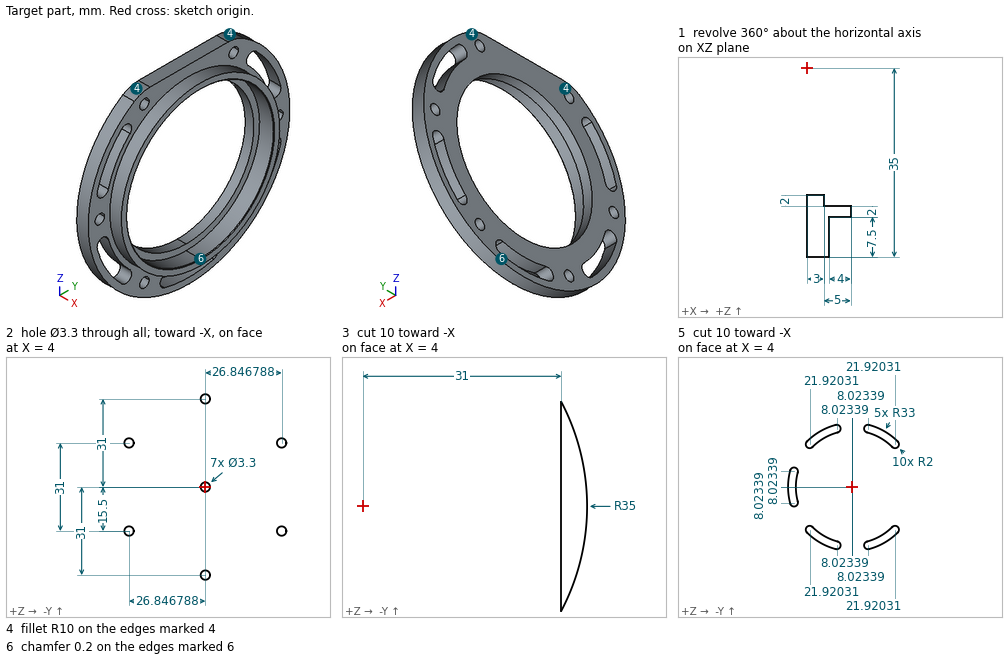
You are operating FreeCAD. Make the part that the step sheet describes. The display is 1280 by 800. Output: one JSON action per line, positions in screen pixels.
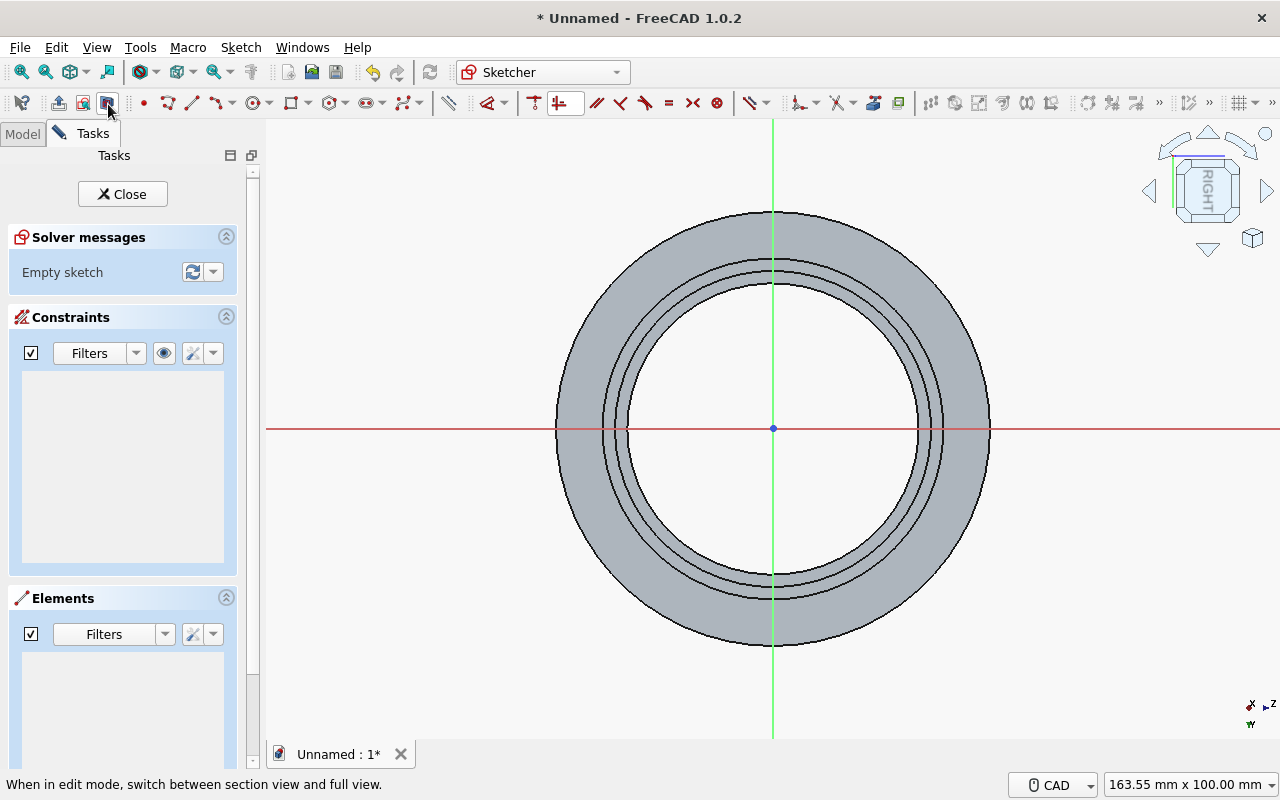
{"action": "left_click", "coordinate": [254, 104]}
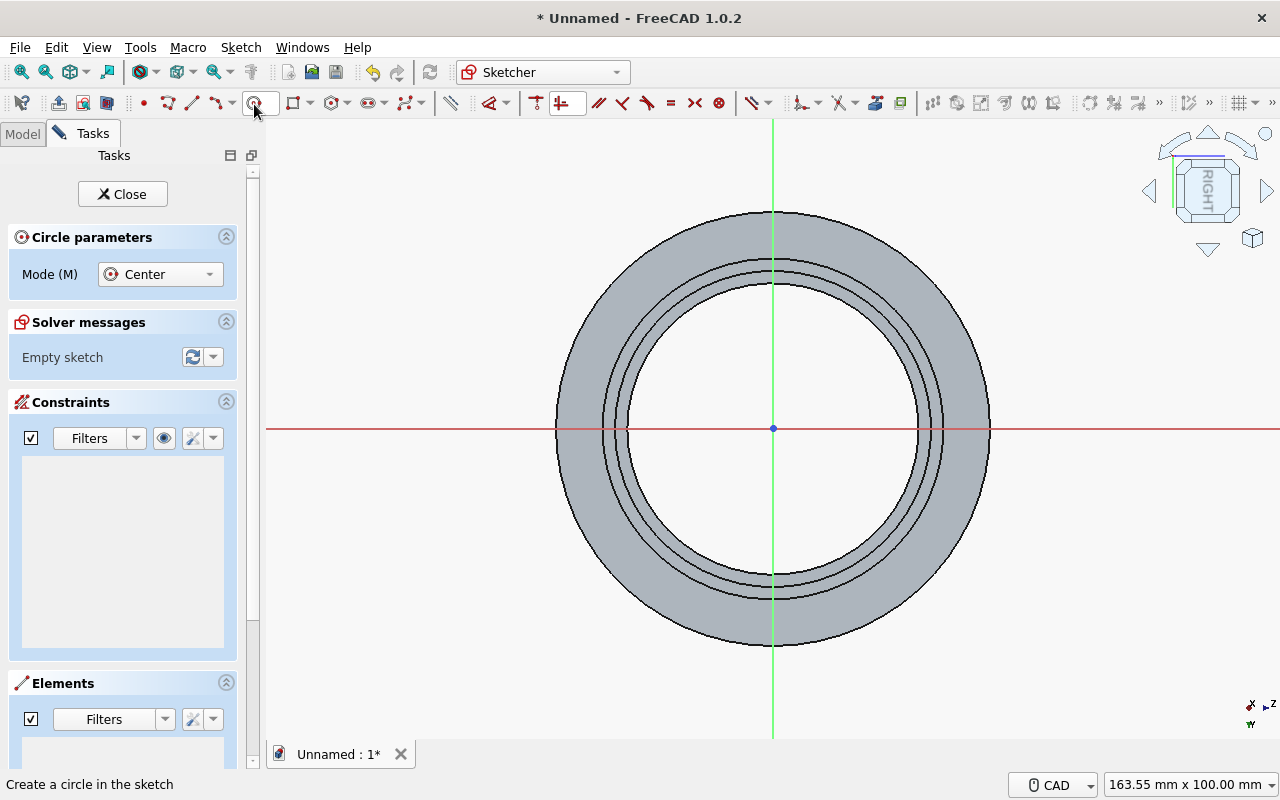
{"action": "scroll", "coordinate": [773, 429], "scroll_direction": "up", "scroll_amount": 4}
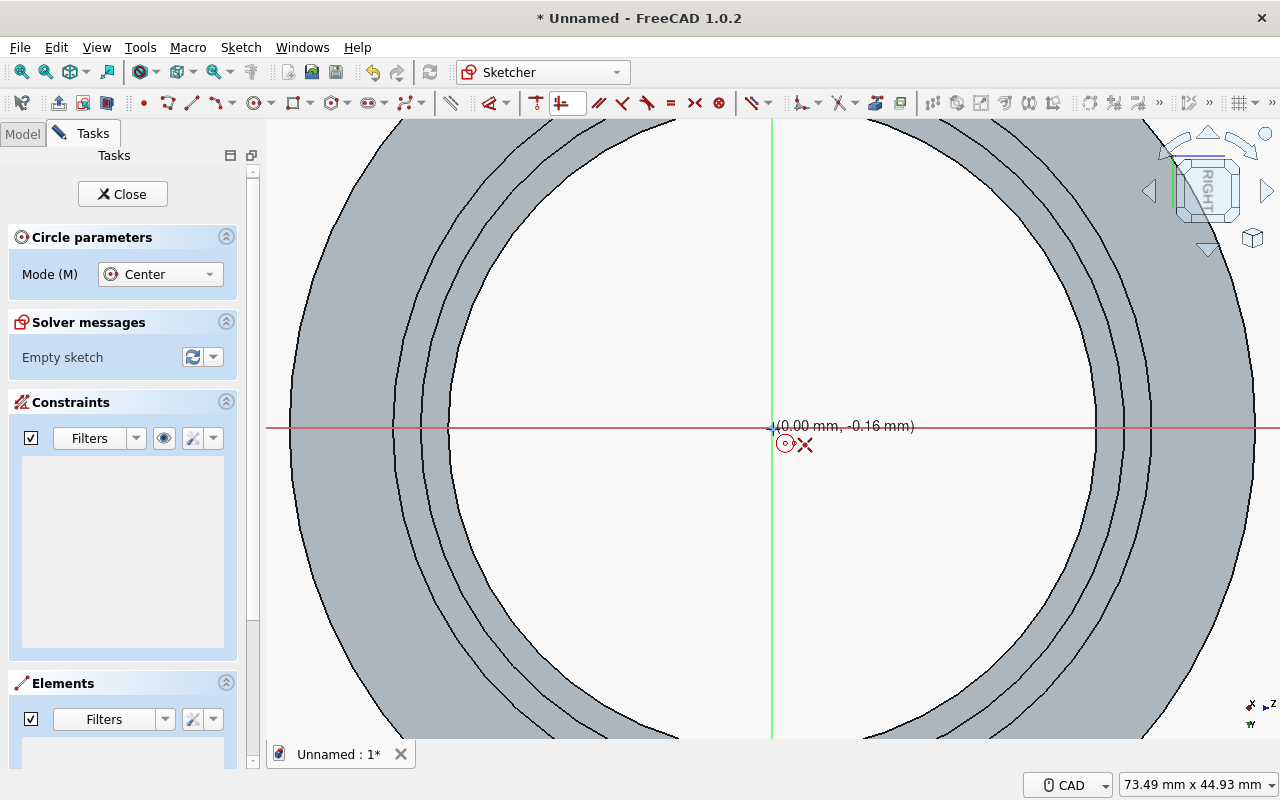
{"action": "left_click", "coordinate": [772, 428]}
{"action": "left_click", "coordinate": [788, 412]}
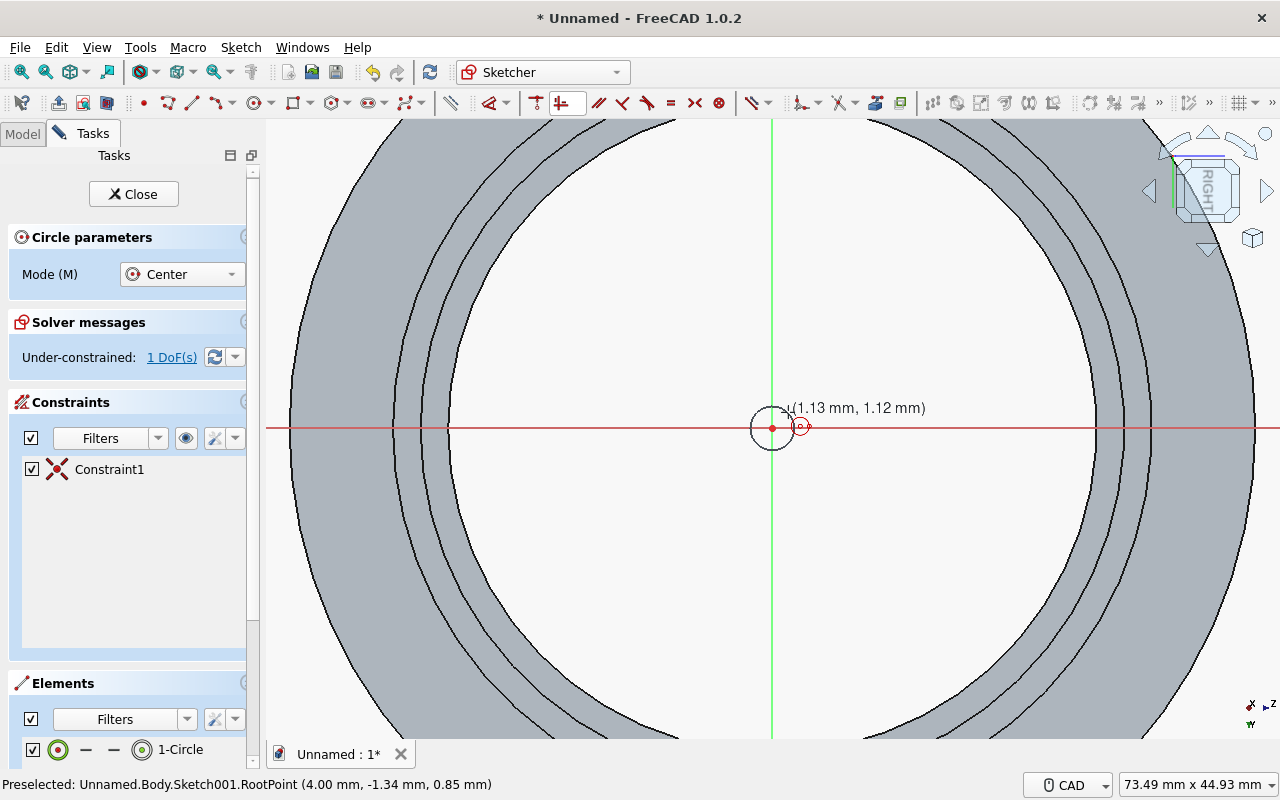
{"action": "scroll", "coordinate": [649, 430], "scroll_direction": "down", "scroll_amount": 4}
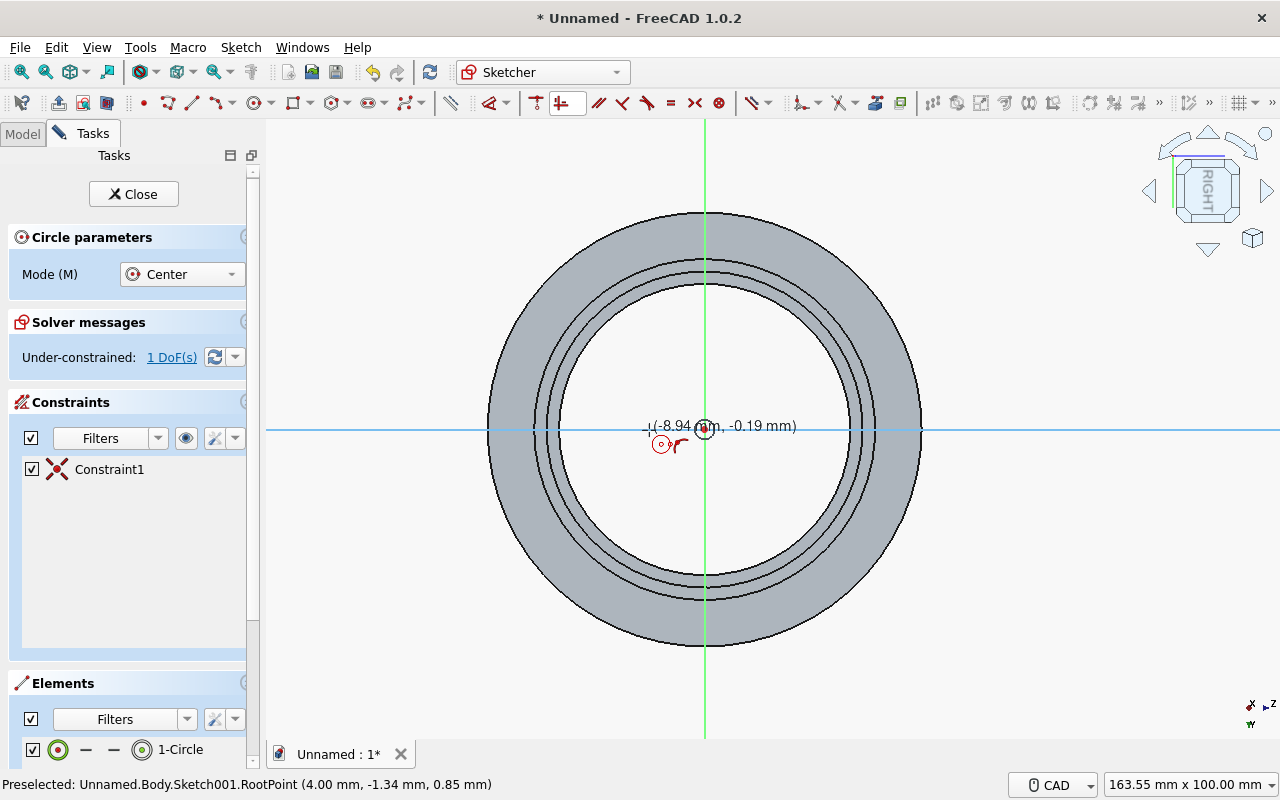
{"action": "scroll", "coordinate": [705, 622], "scroll_direction": "up", "scroll_amount": 4}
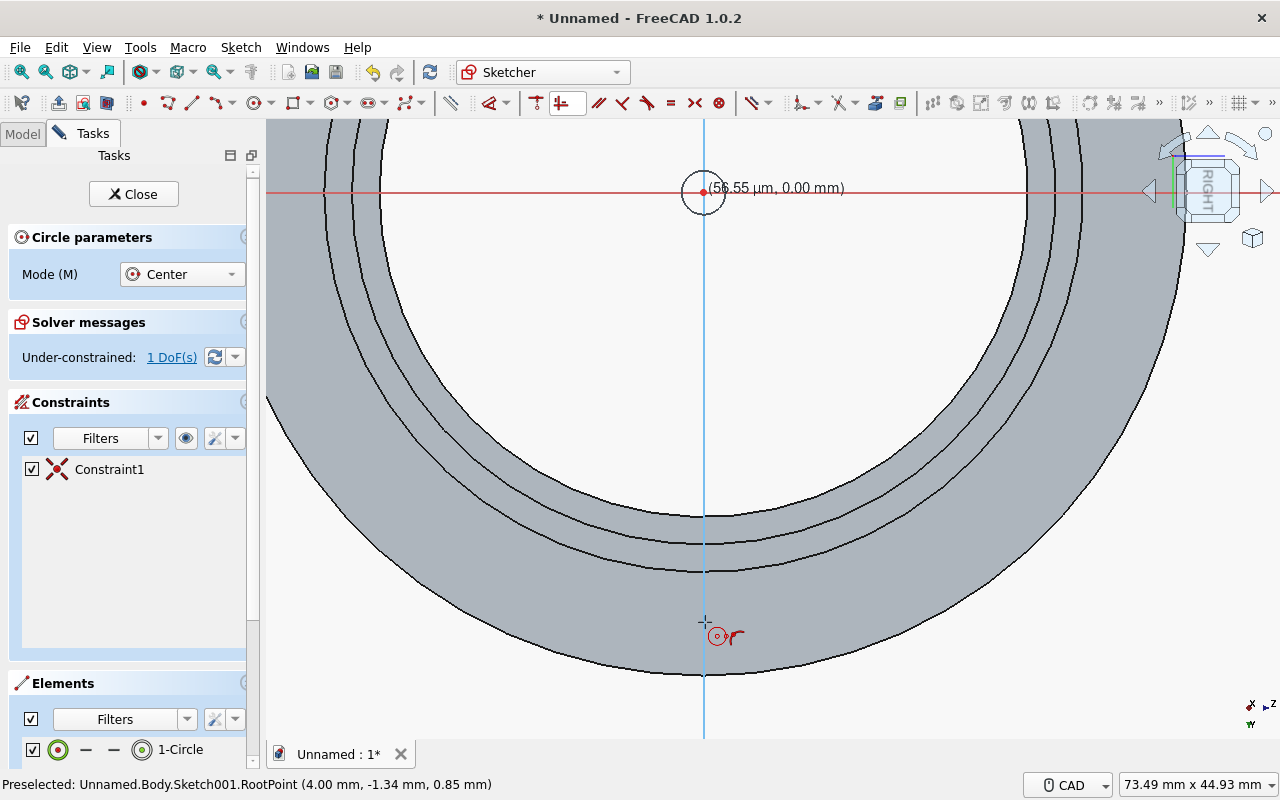
{"action": "left_click", "coordinate": [704, 620]}
{"action": "left_click", "coordinate": [720, 604]}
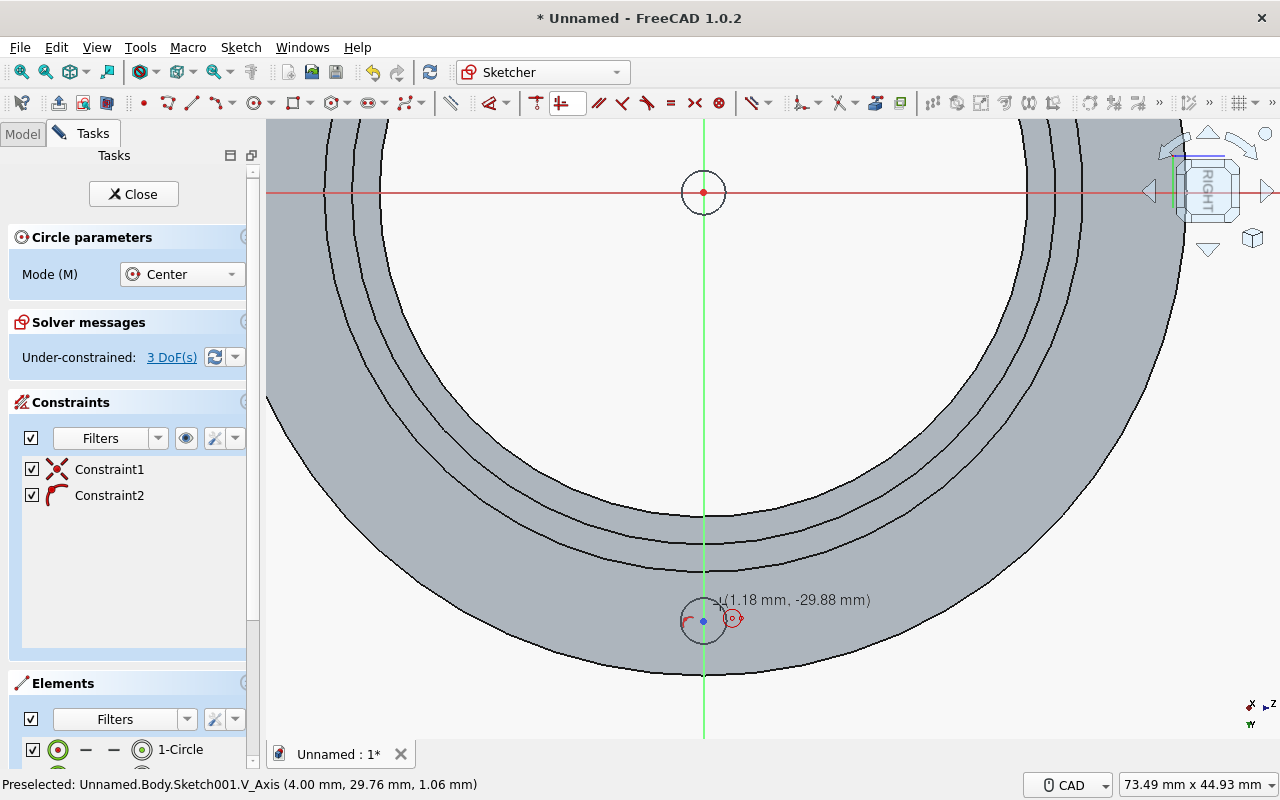
{"action": "left_click", "coordinate": [333, 407]}
{"action": "left_click", "coordinate": [349, 390]}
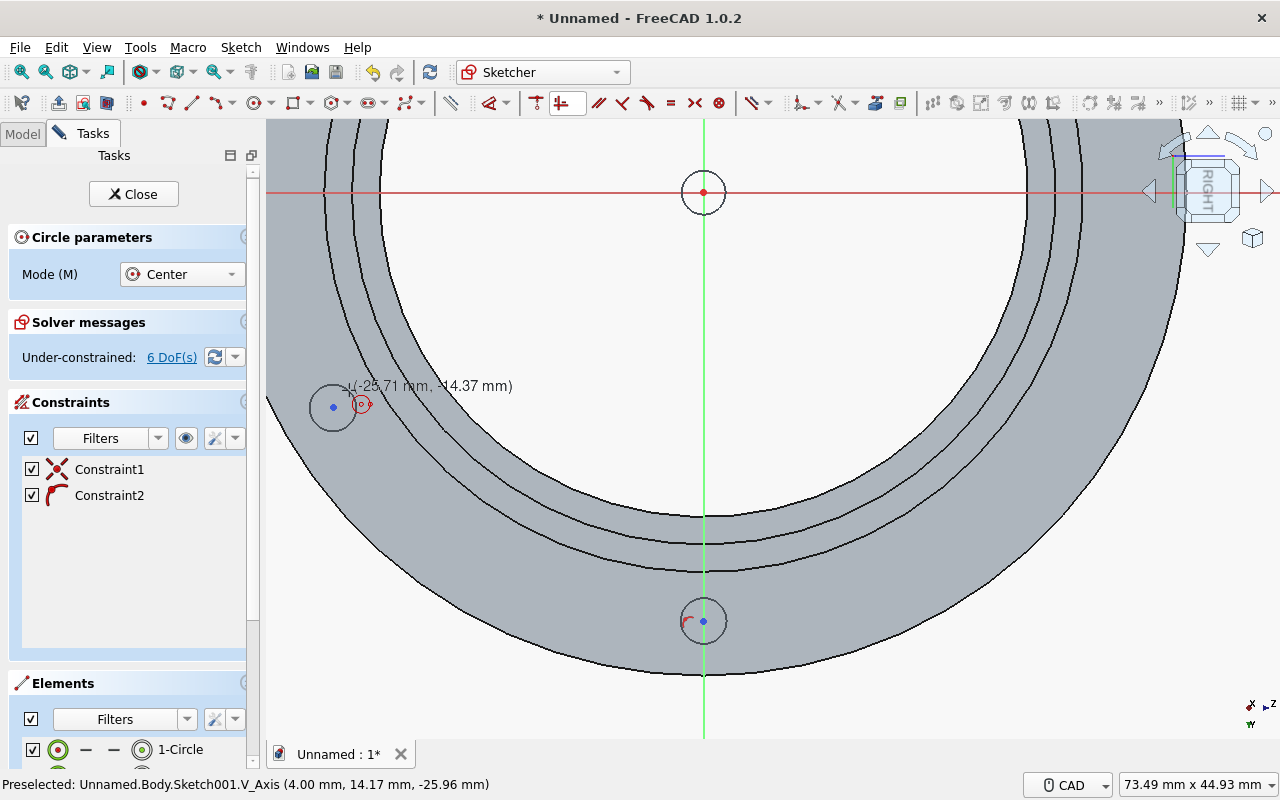
{"action": "scroll", "coordinate": [705, 622], "scroll_direction": "down", "scroll_amount": 4}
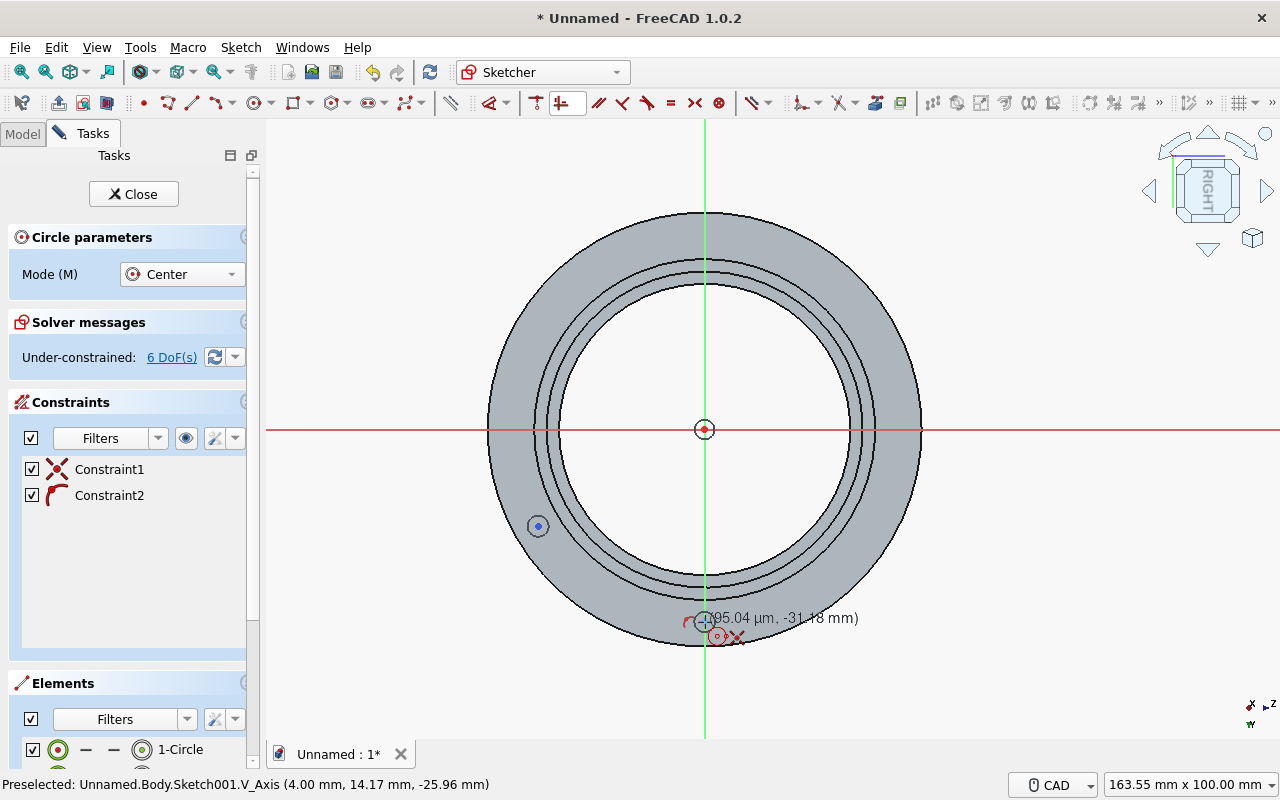
{"action": "scroll", "coordinate": [538, 333], "scroll_direction": "up", "scroll_amount": 4}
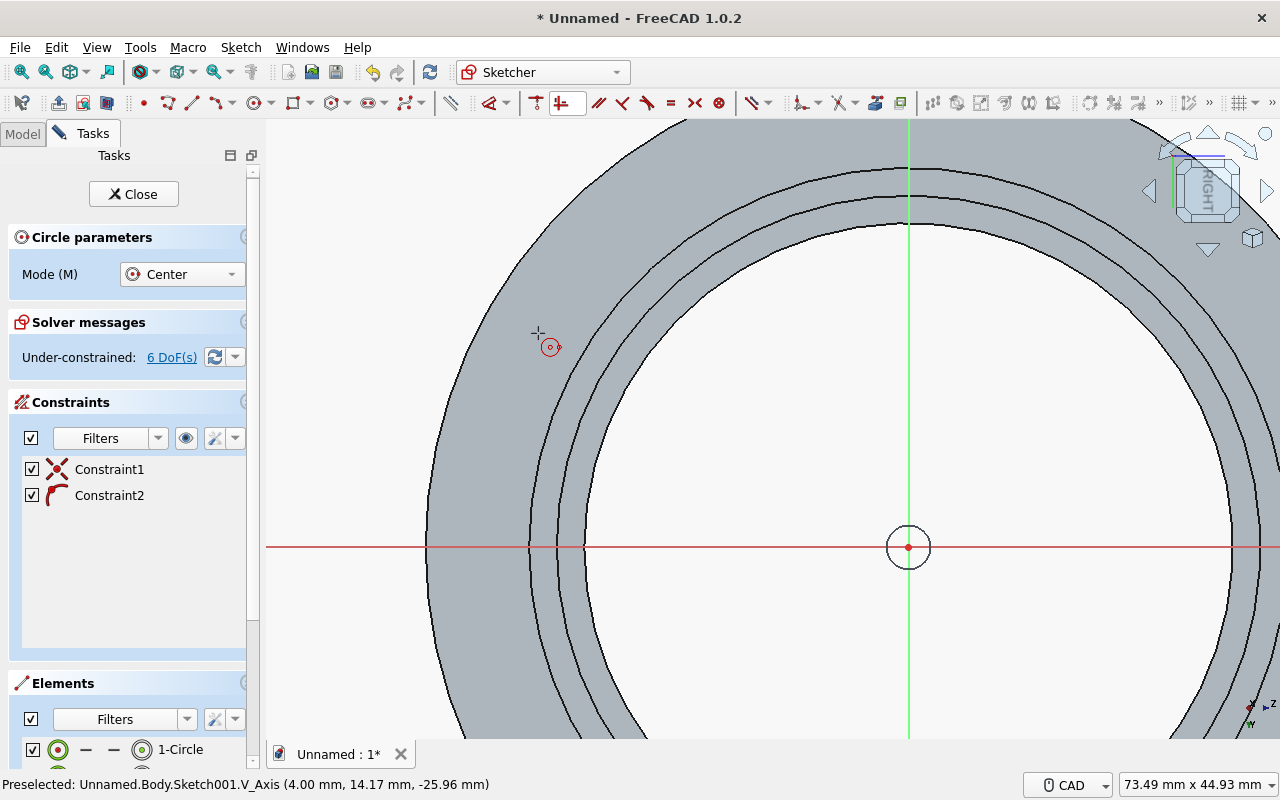
{"action": "left_click", "coordinate": [538, 334]}
{"action": "left_click", "coordinate": [554, 317]}